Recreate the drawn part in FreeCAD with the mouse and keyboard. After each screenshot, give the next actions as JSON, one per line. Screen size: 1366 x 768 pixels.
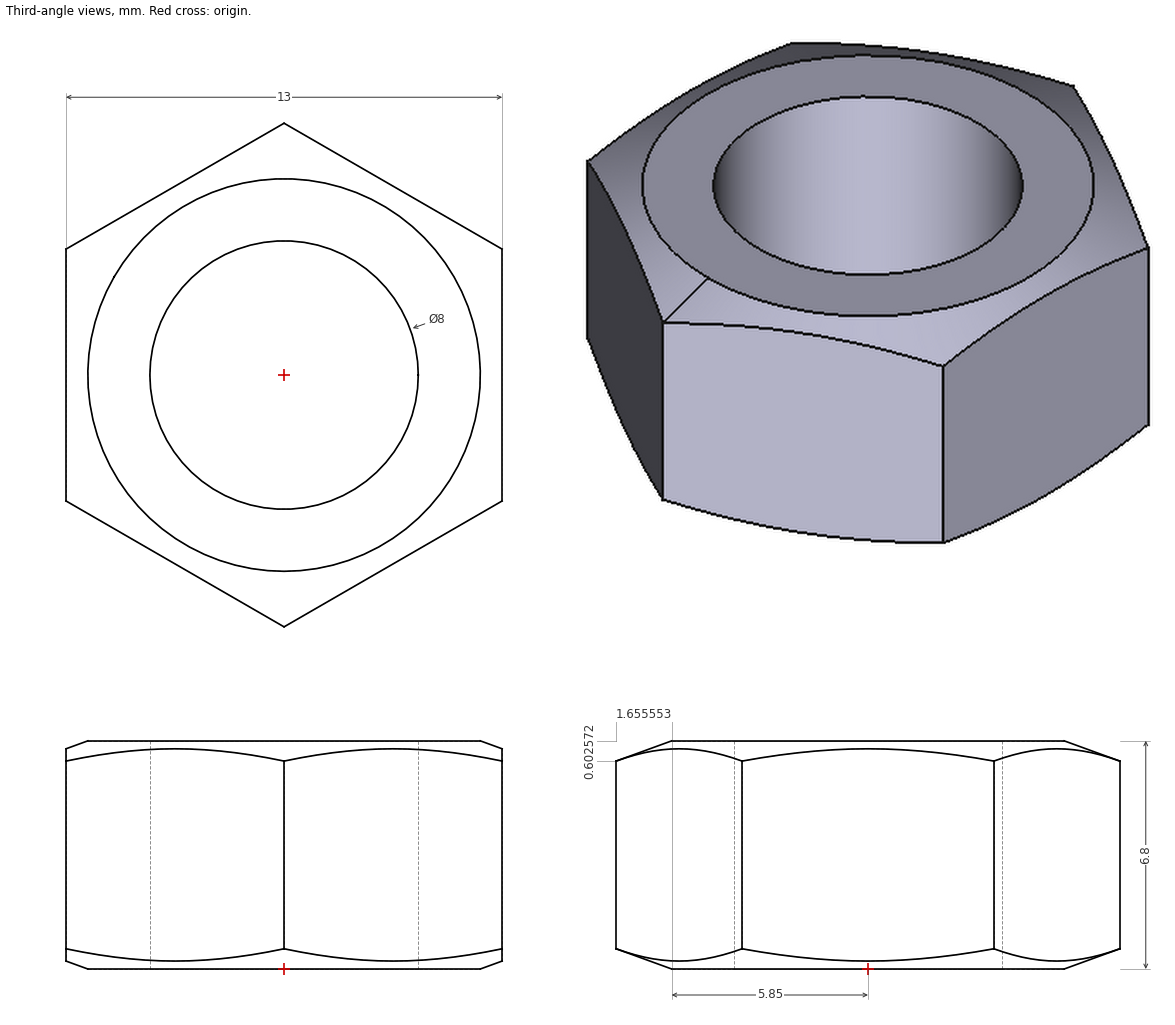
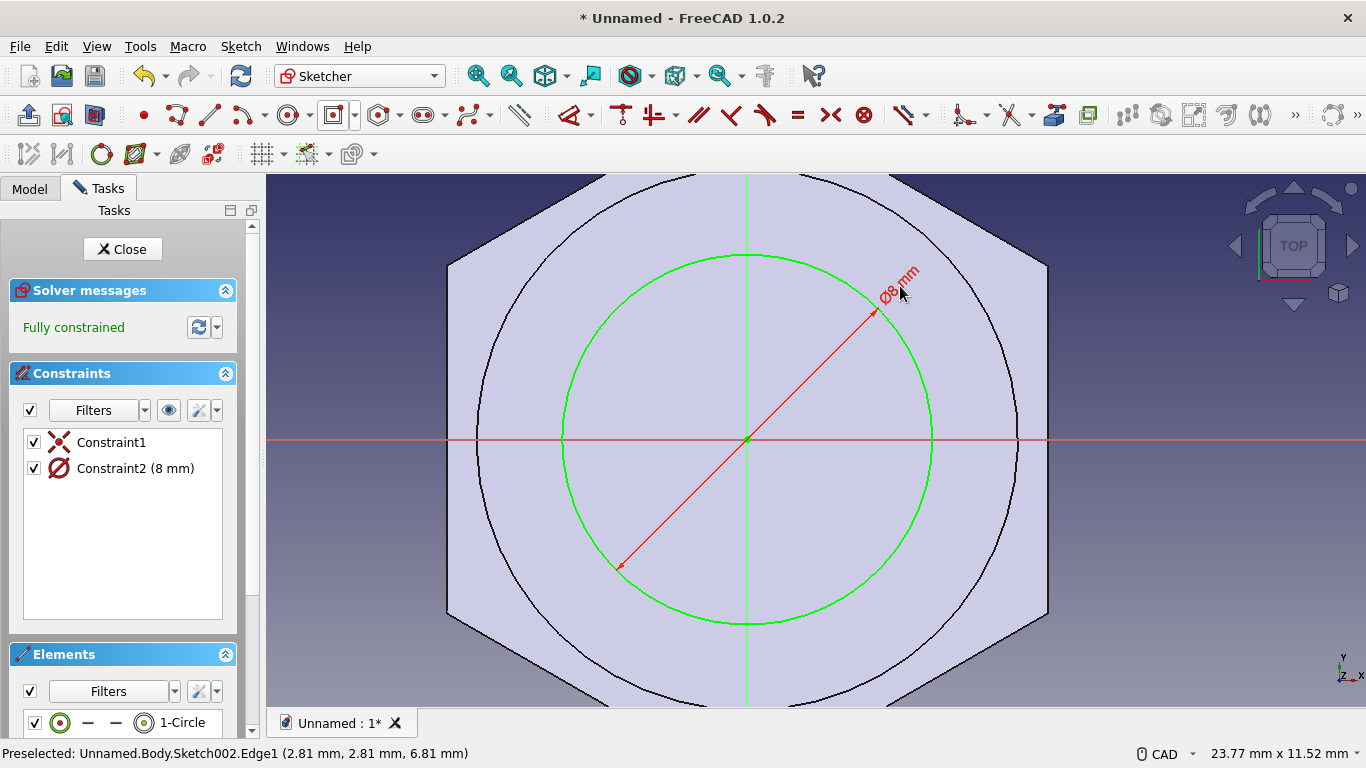
{"action": "left_click", "coordinate": [123, 249]}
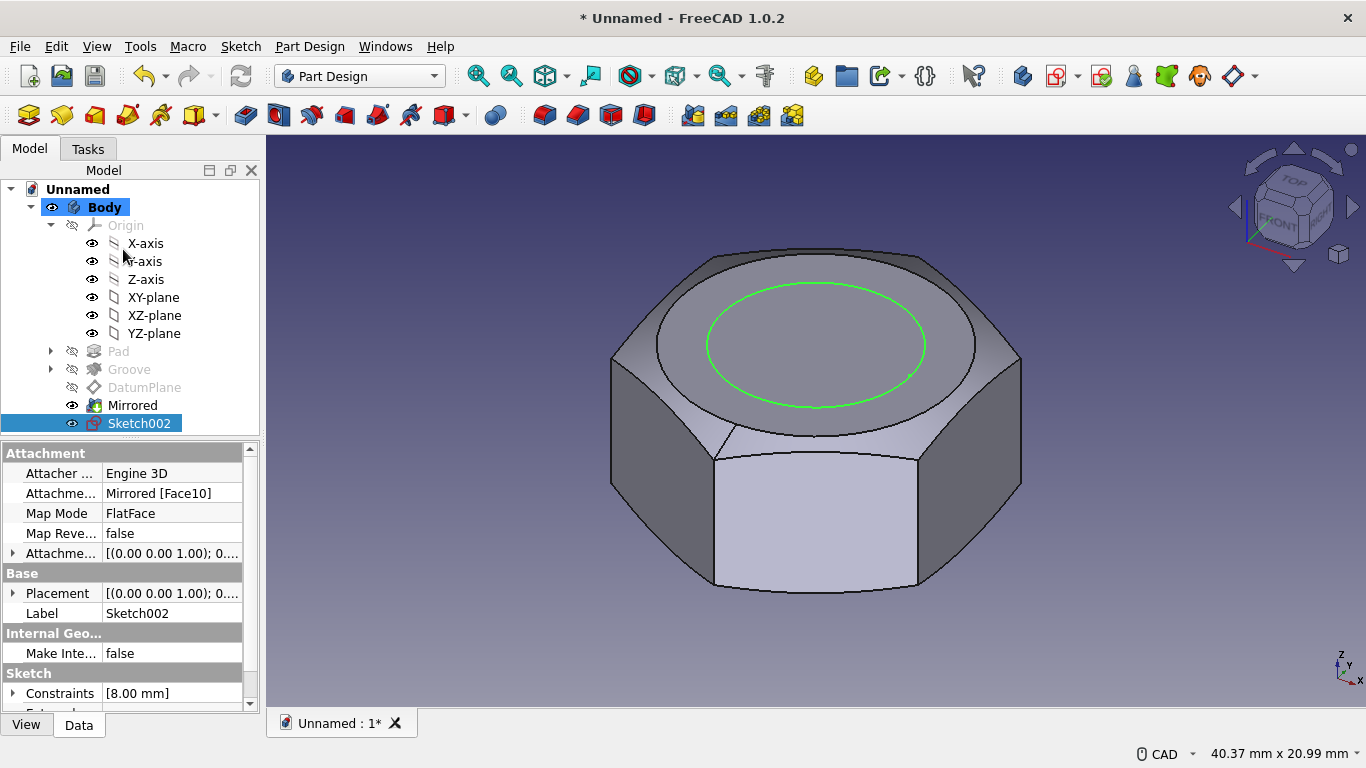
{"action": "left_click", "coordinate": [246, 116]}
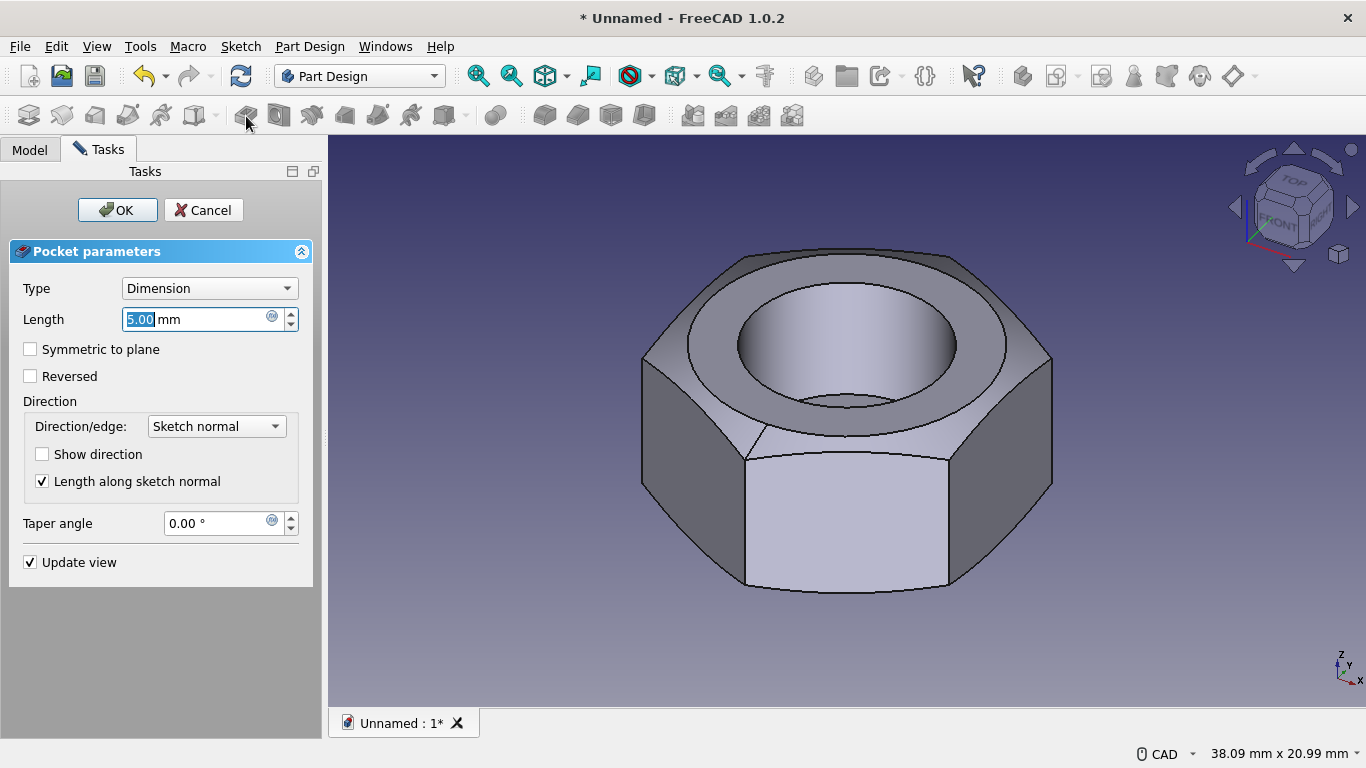
{"action": "left_click", "coordinate": [210, 288]}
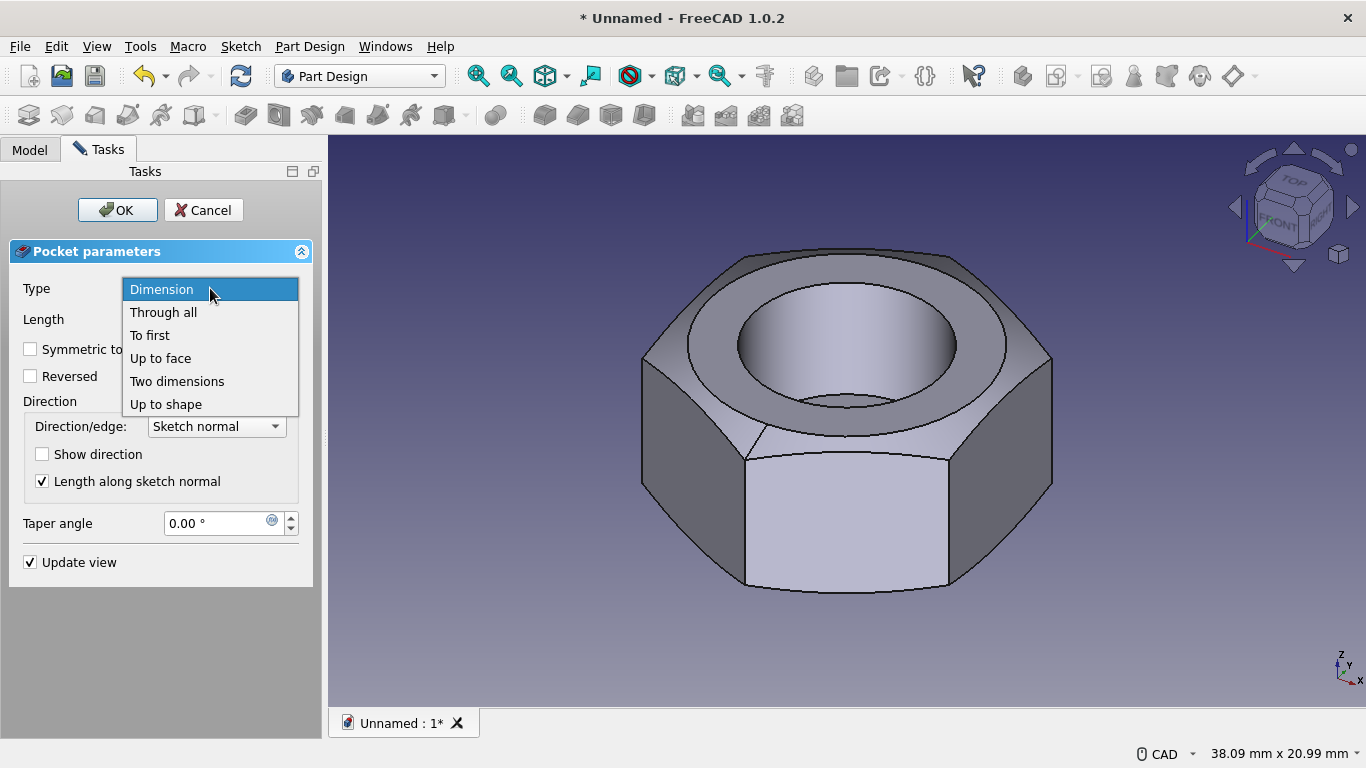
{"action": "left_click", "coordinate": [208, 312]}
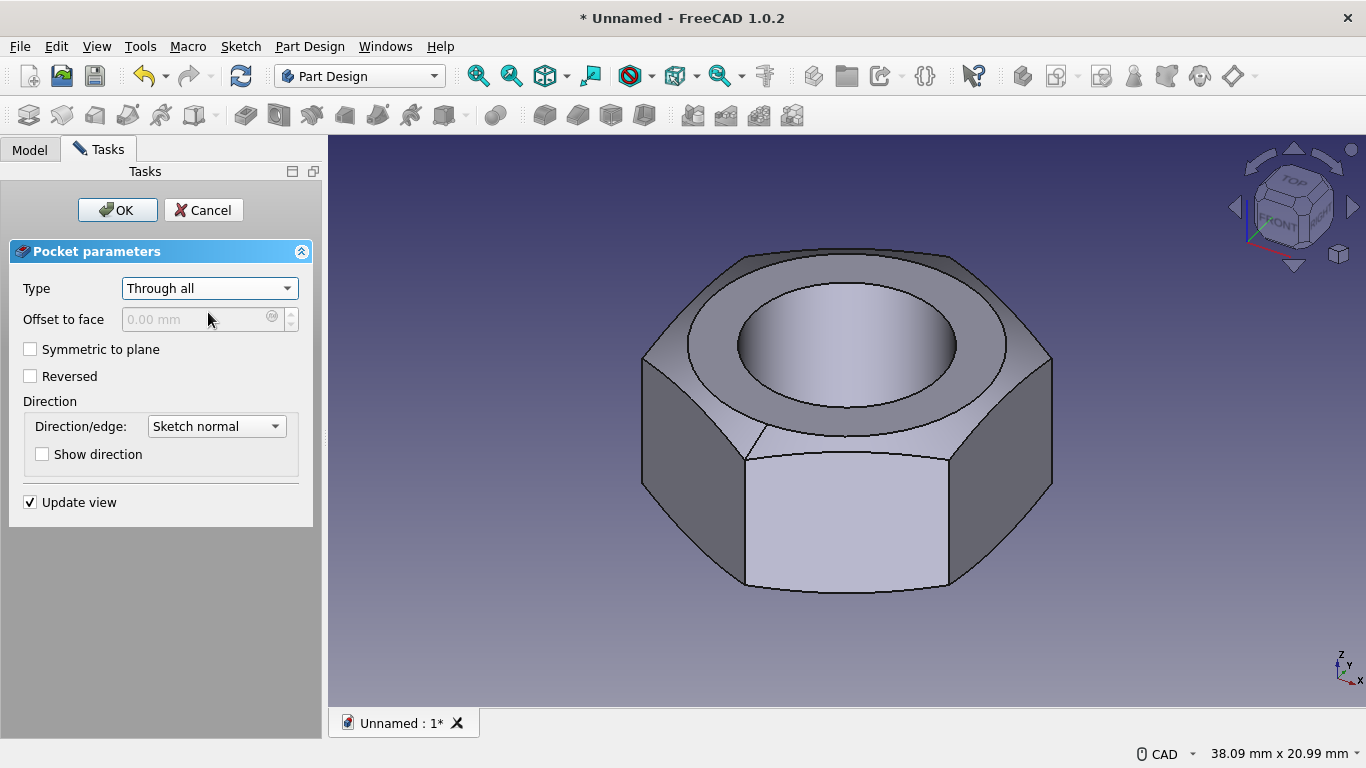
{"action": "left_click", "coordinate": [118, 210]}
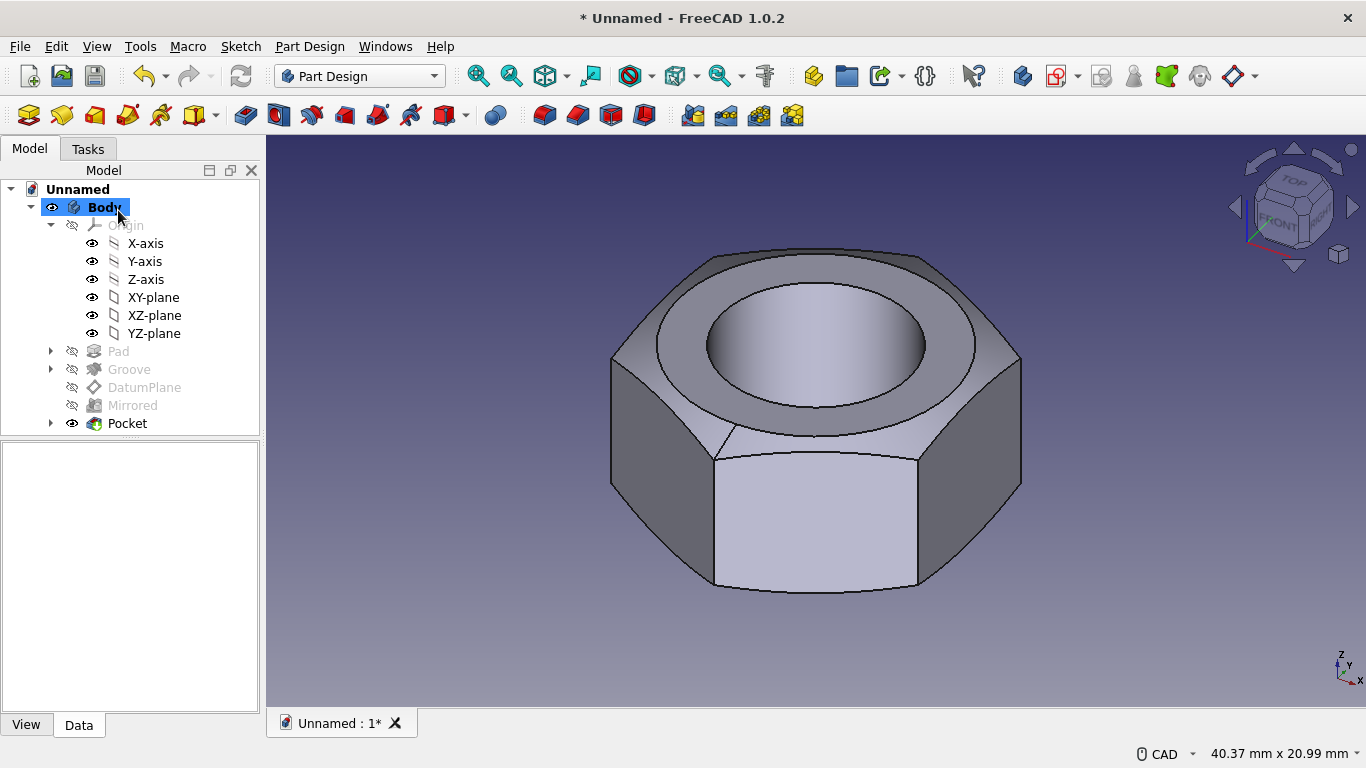
{"action": "key", "text": "0"}